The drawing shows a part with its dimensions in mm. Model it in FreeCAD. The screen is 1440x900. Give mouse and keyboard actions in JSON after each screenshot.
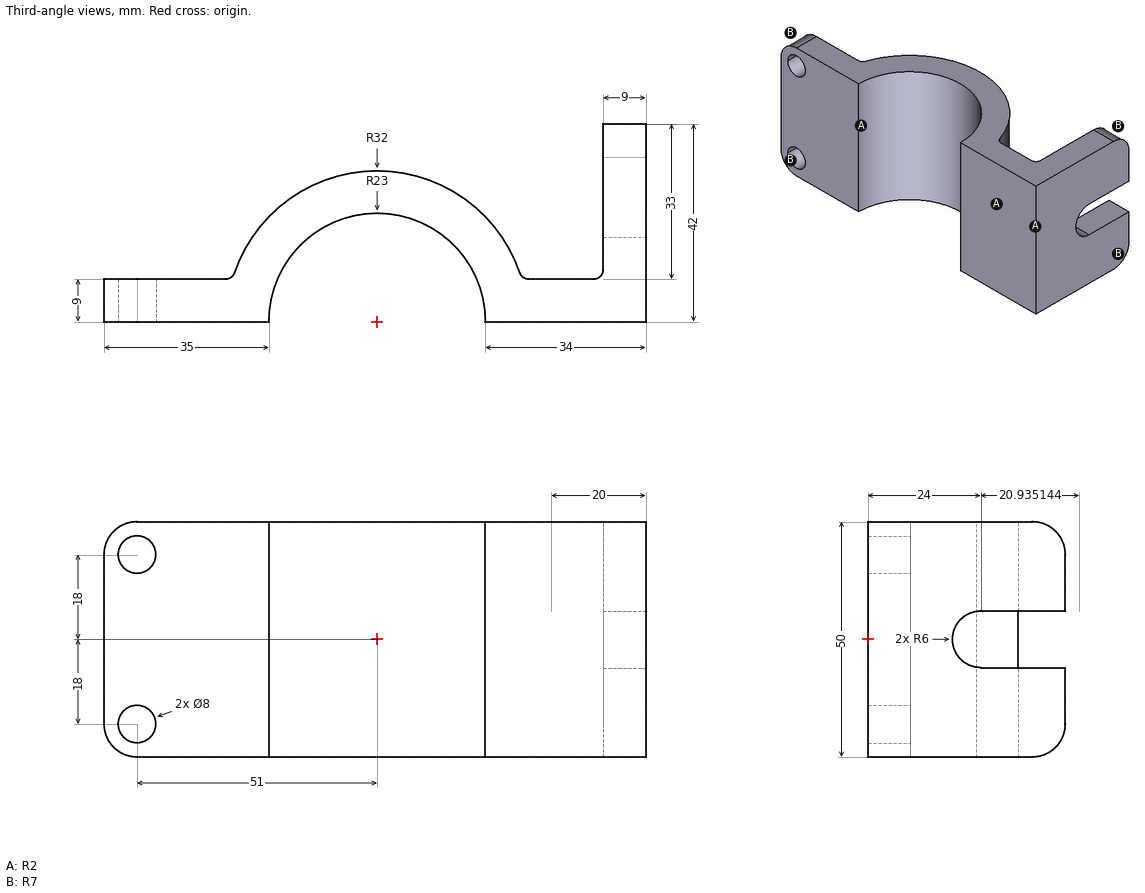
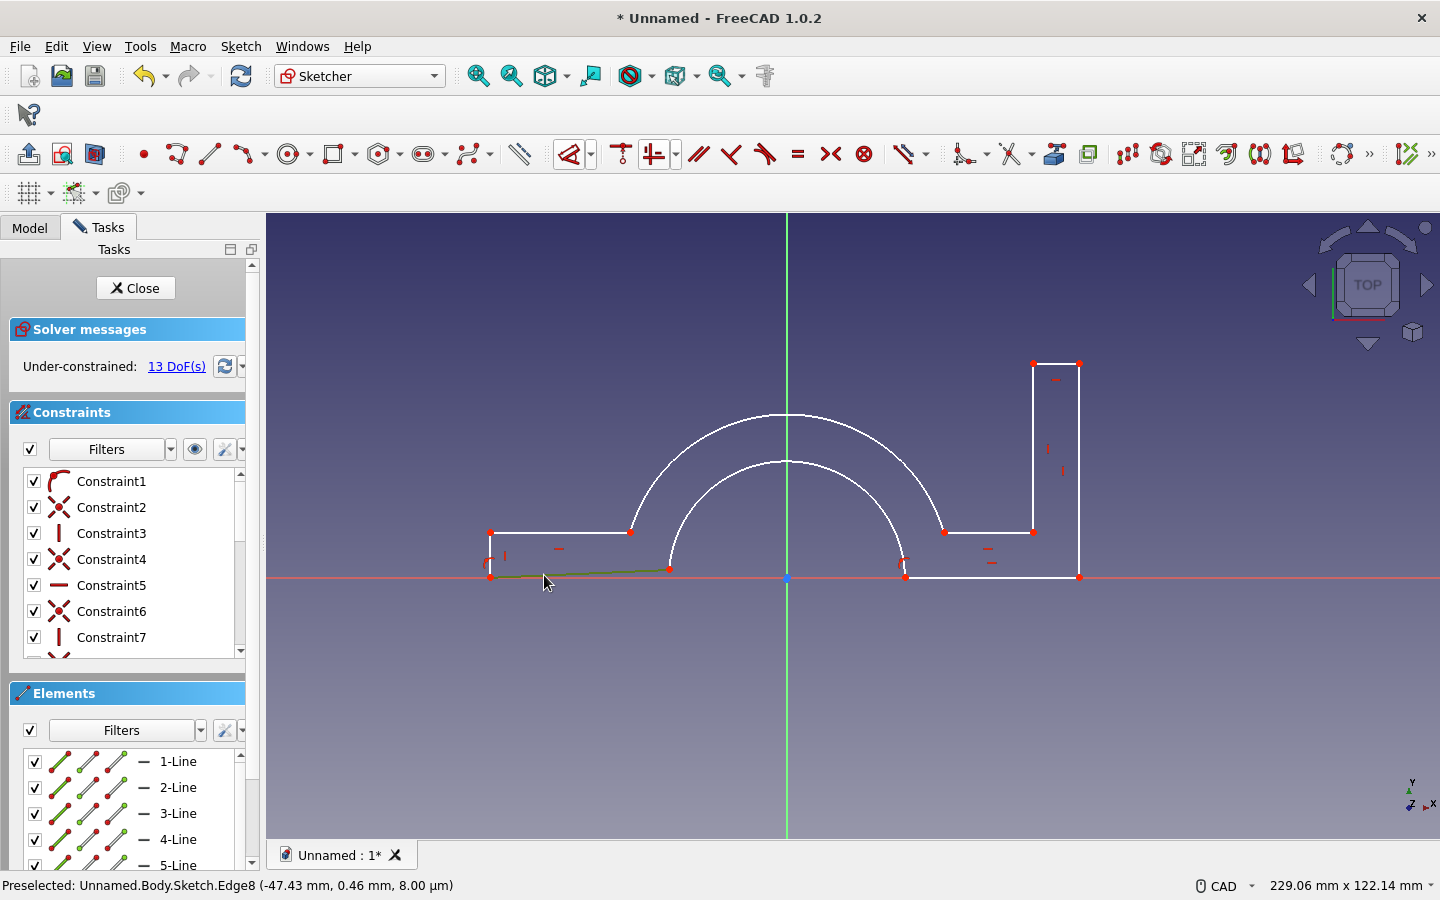
{"action": "left_click", "coordinate": [676, 154]}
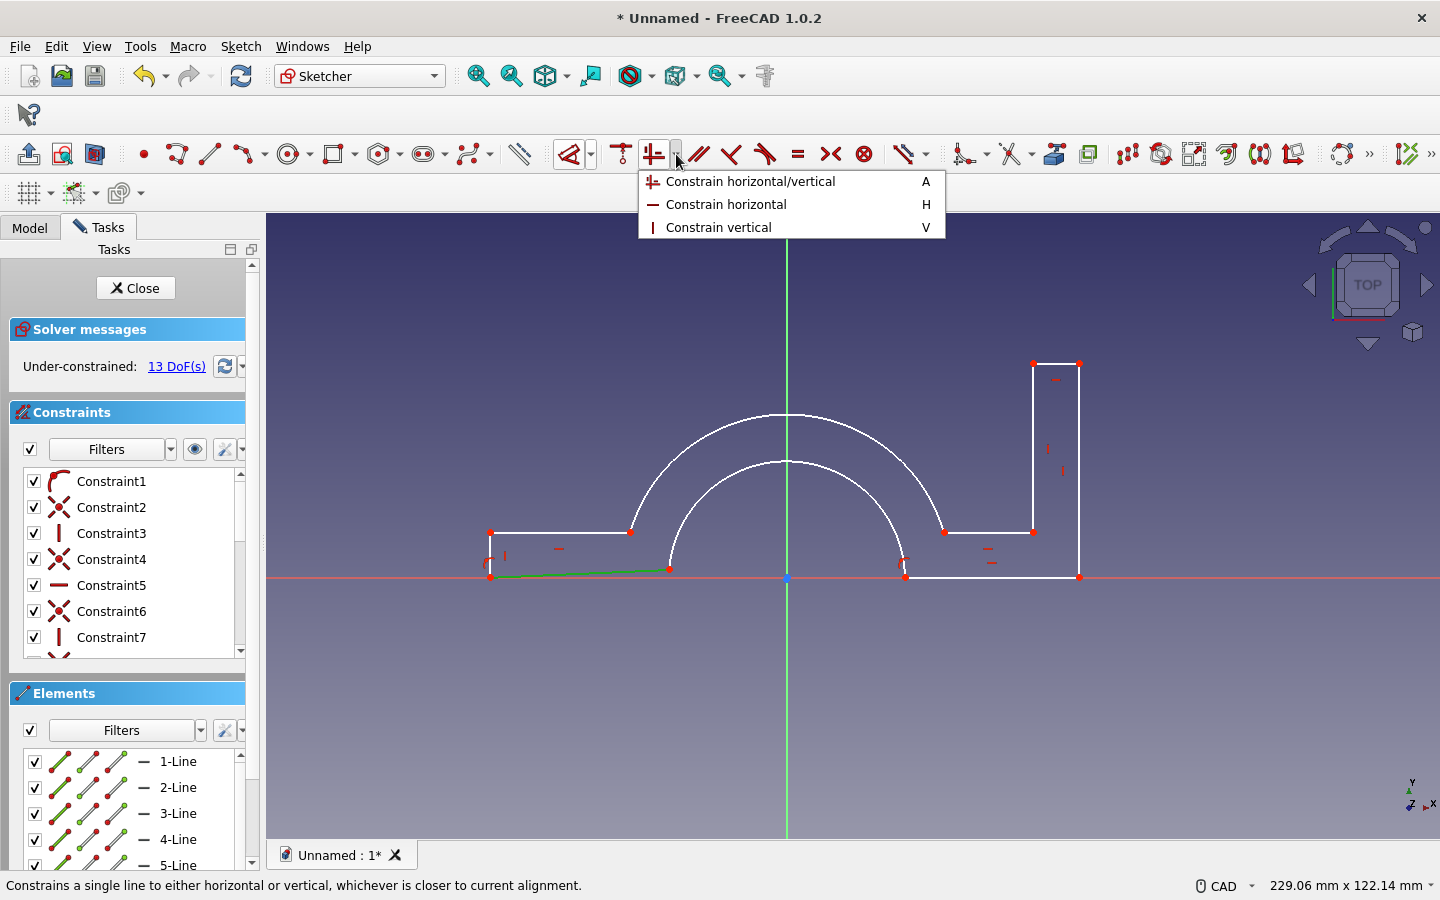
{"action": "left_click", "coordinate": [792, 204]}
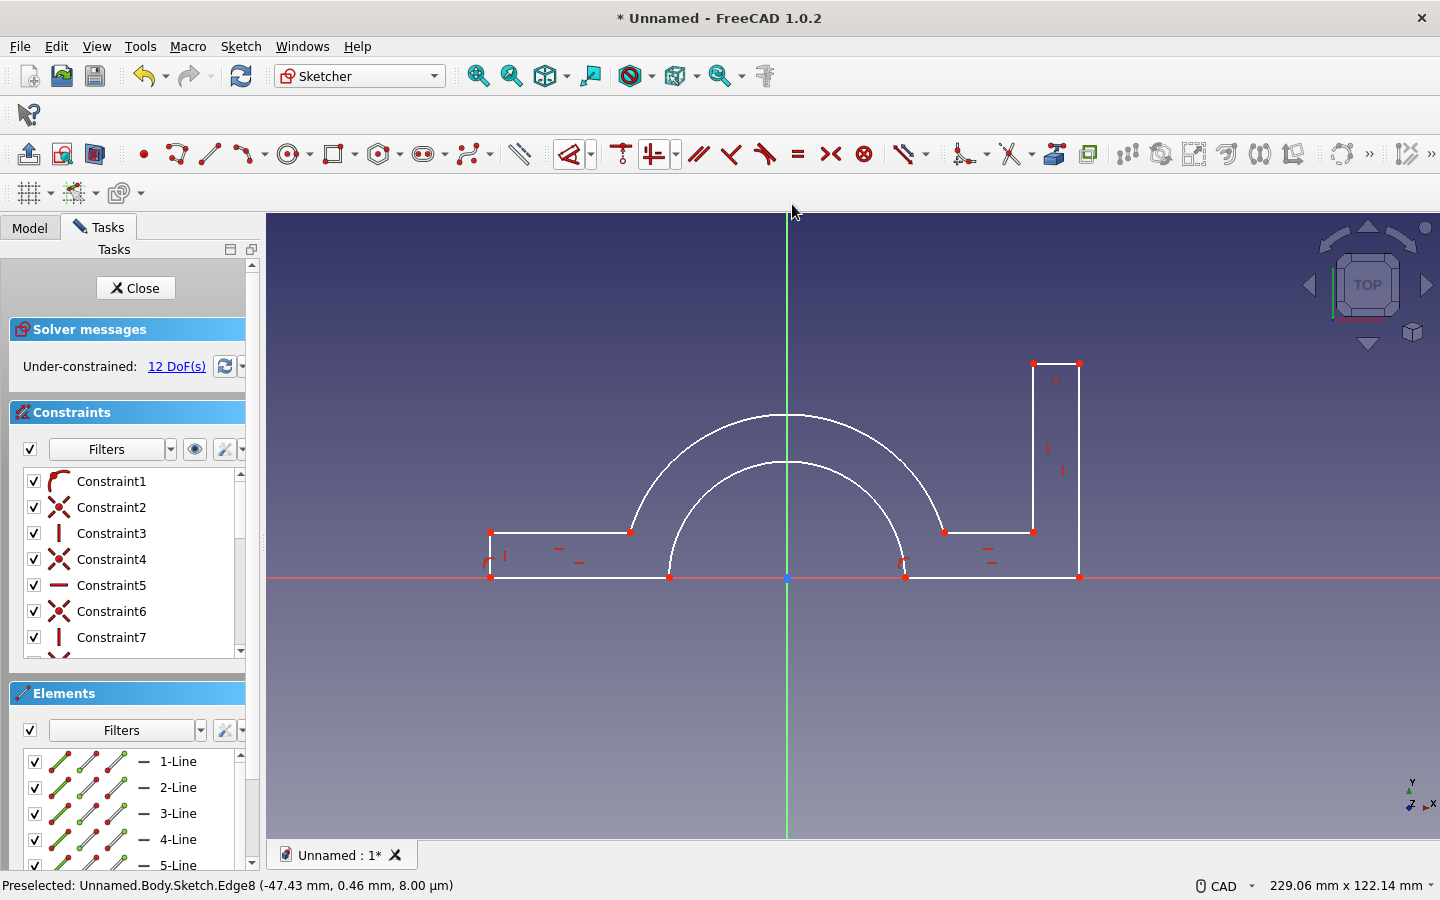
{"action": "left_click", "coordinate": [868, 436]}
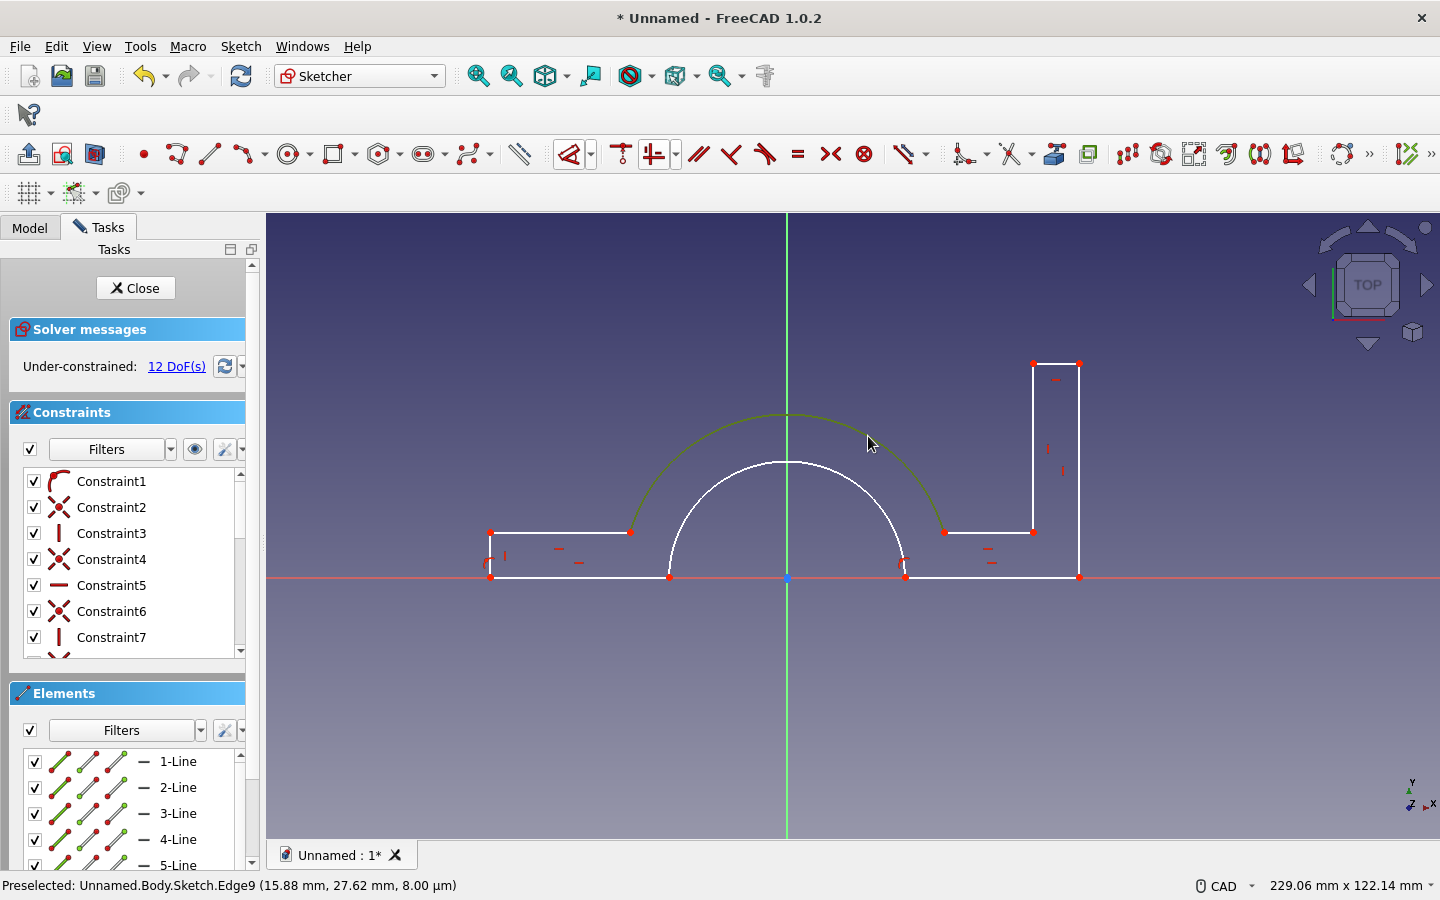
{"action": "left_click", "coordinate": [856, 484]}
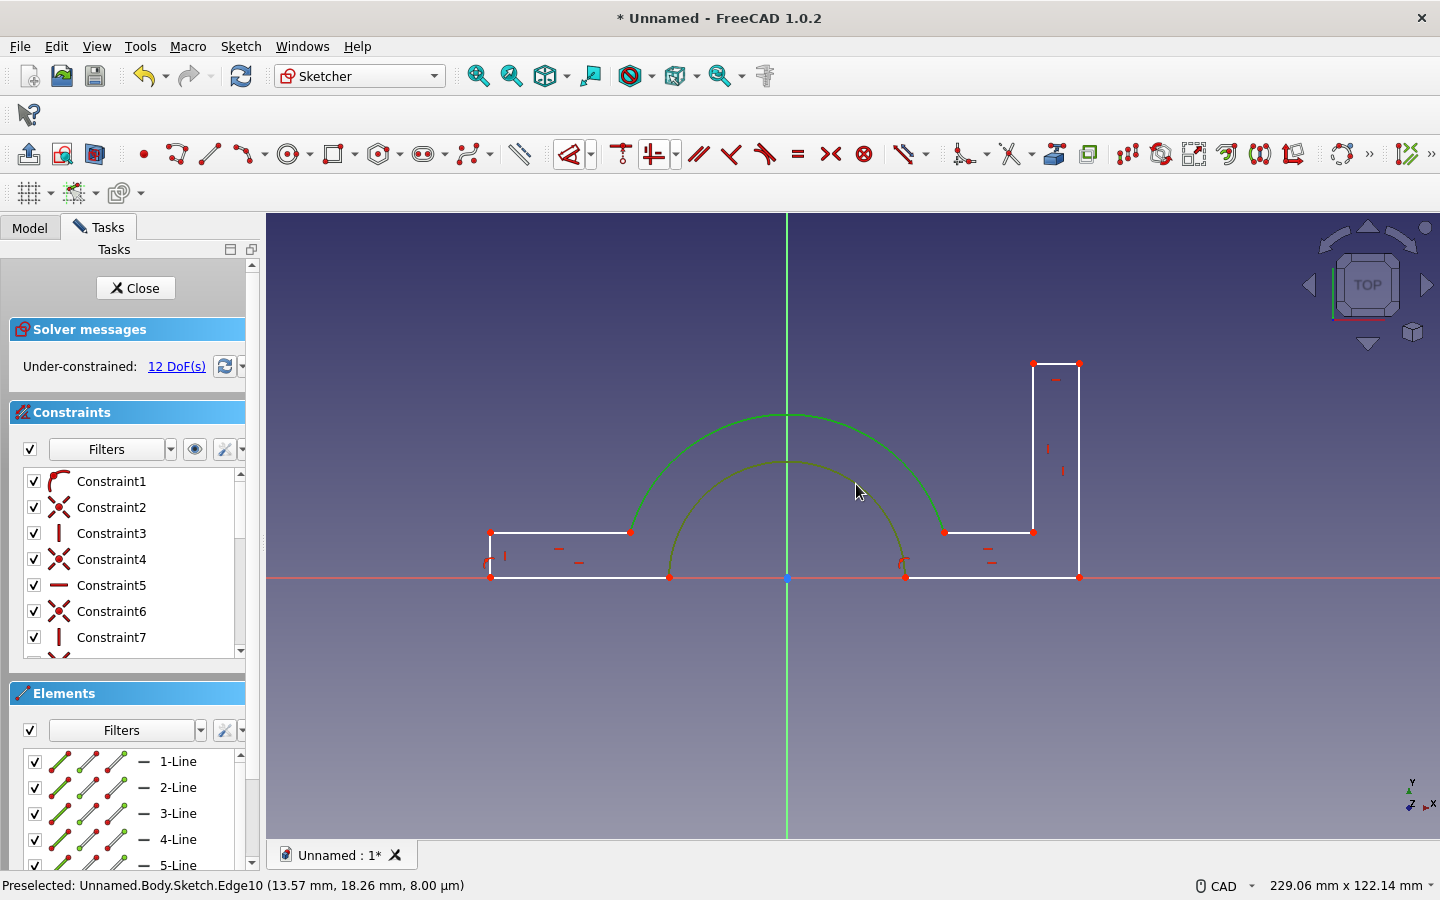
{"action": "left_click", "coordinate": [621, 154]}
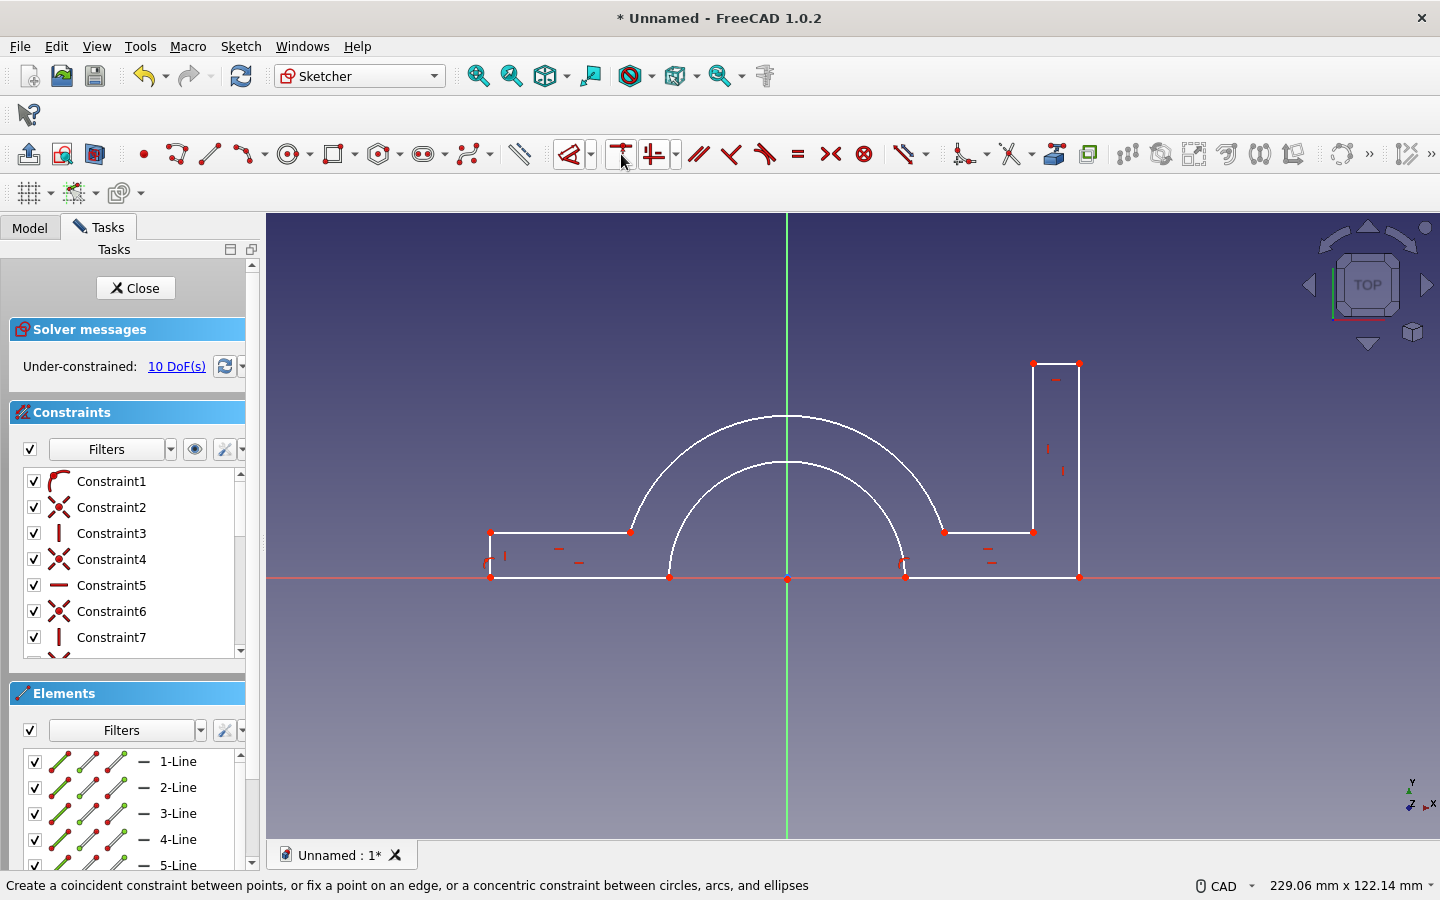
{"action": "left_click_drag", "start_coordinate": [777, 568], "coordinate": [797, 590]}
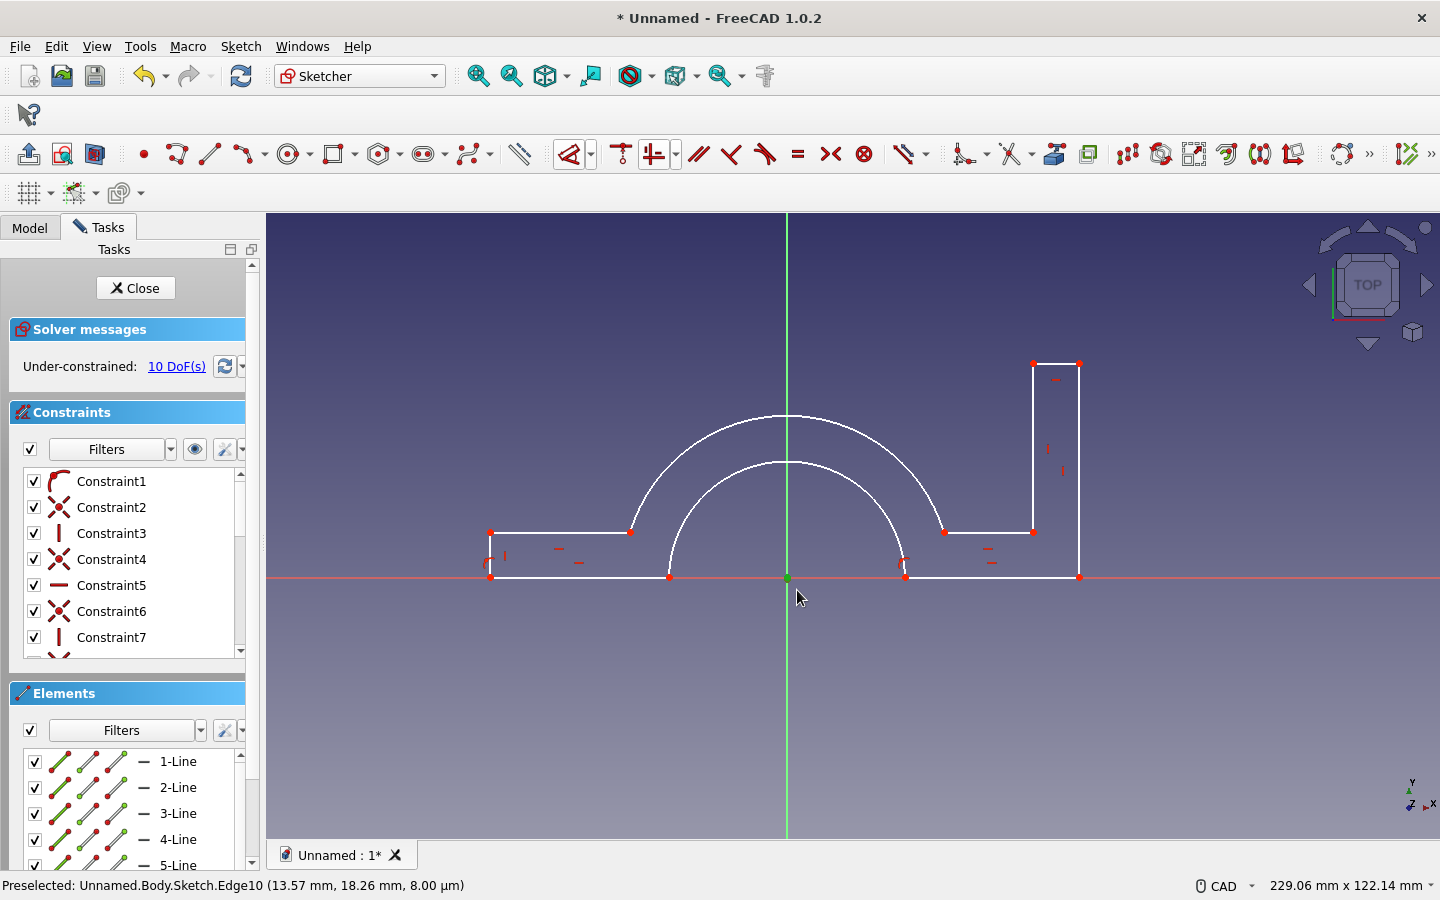
{"action": "left_click", "coordinate": [621, 154]}